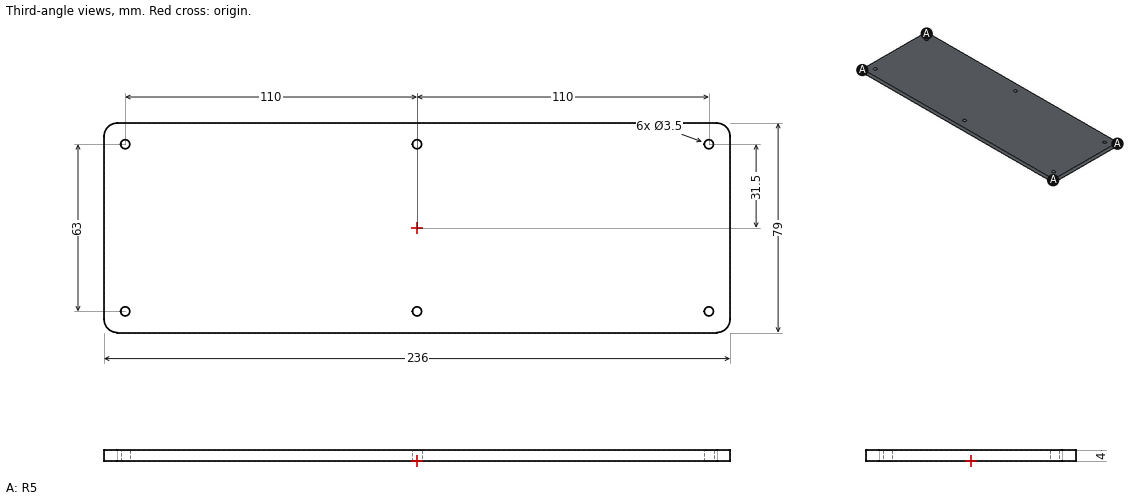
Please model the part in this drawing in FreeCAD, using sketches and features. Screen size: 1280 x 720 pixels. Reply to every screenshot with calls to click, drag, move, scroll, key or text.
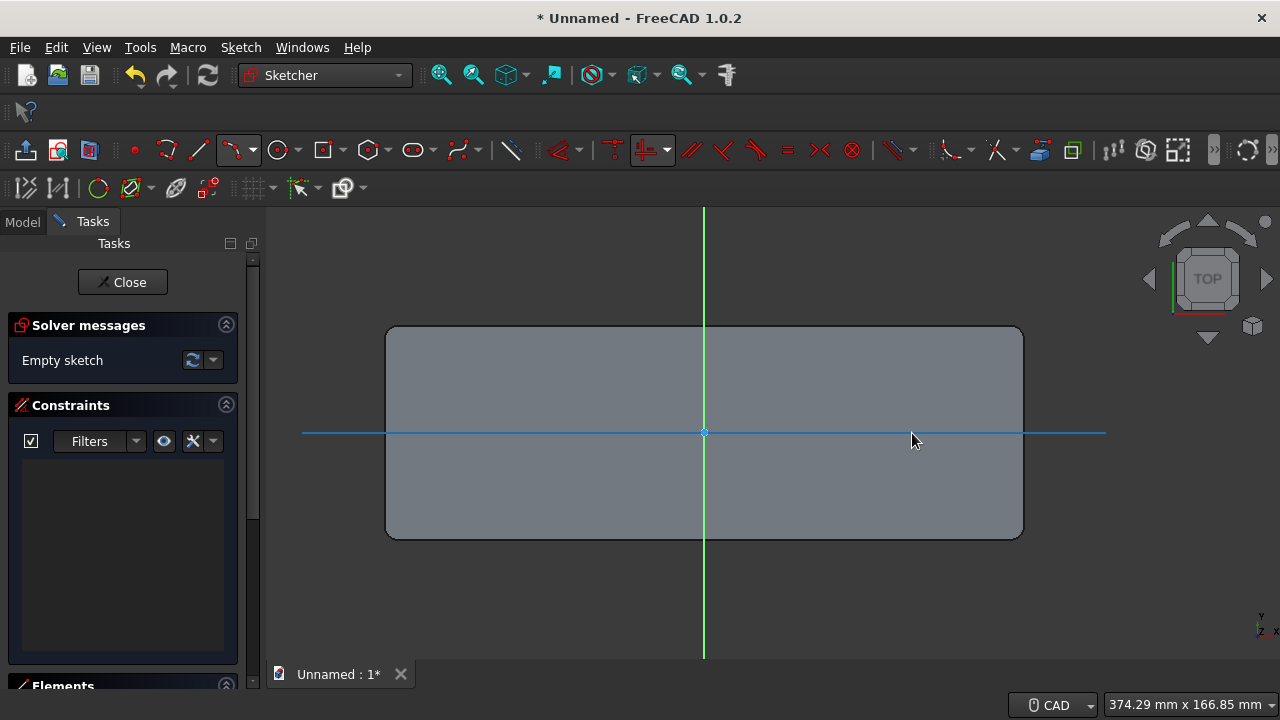
click(278, 150)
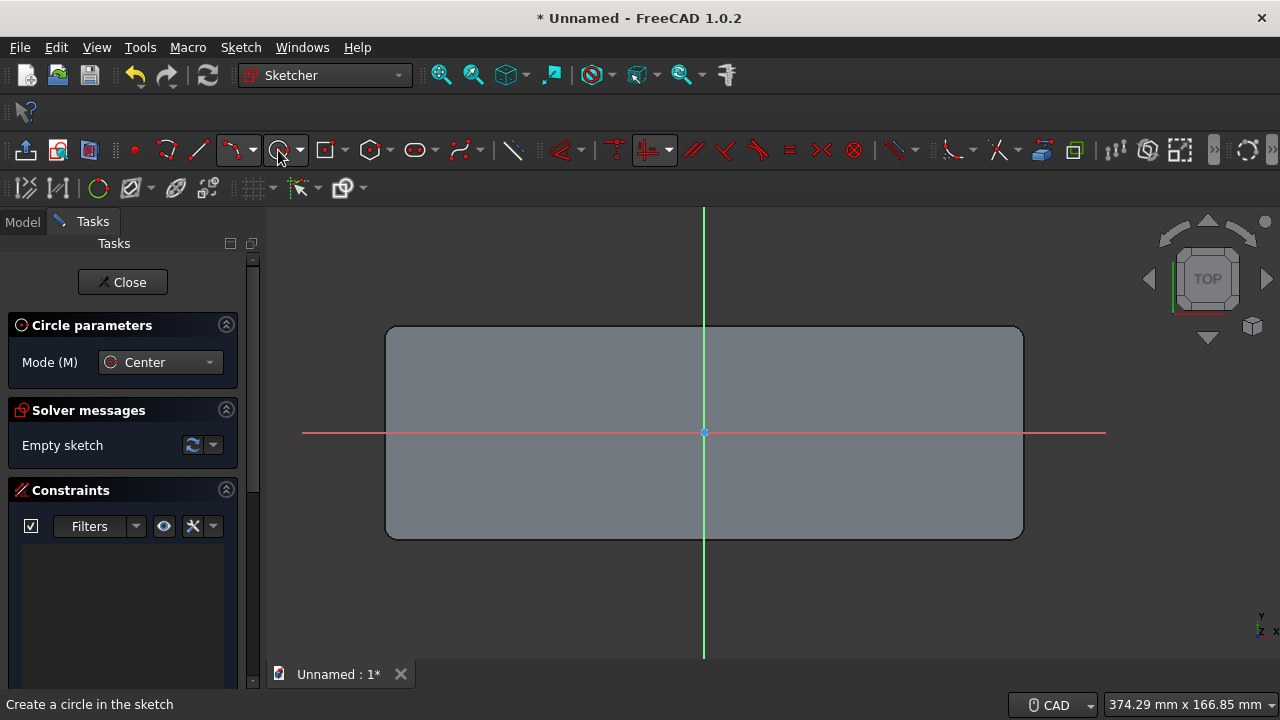
scroll(1002, 347, up, 8)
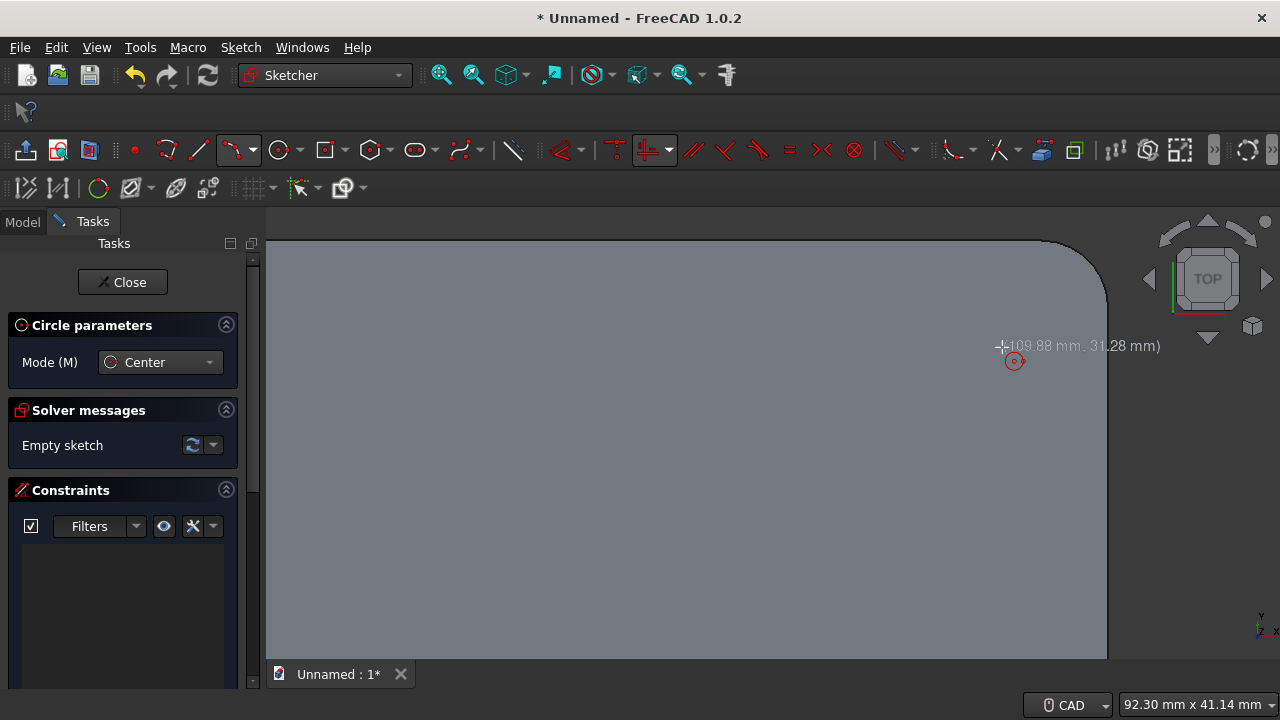
scroll(1003, 348, down, 8)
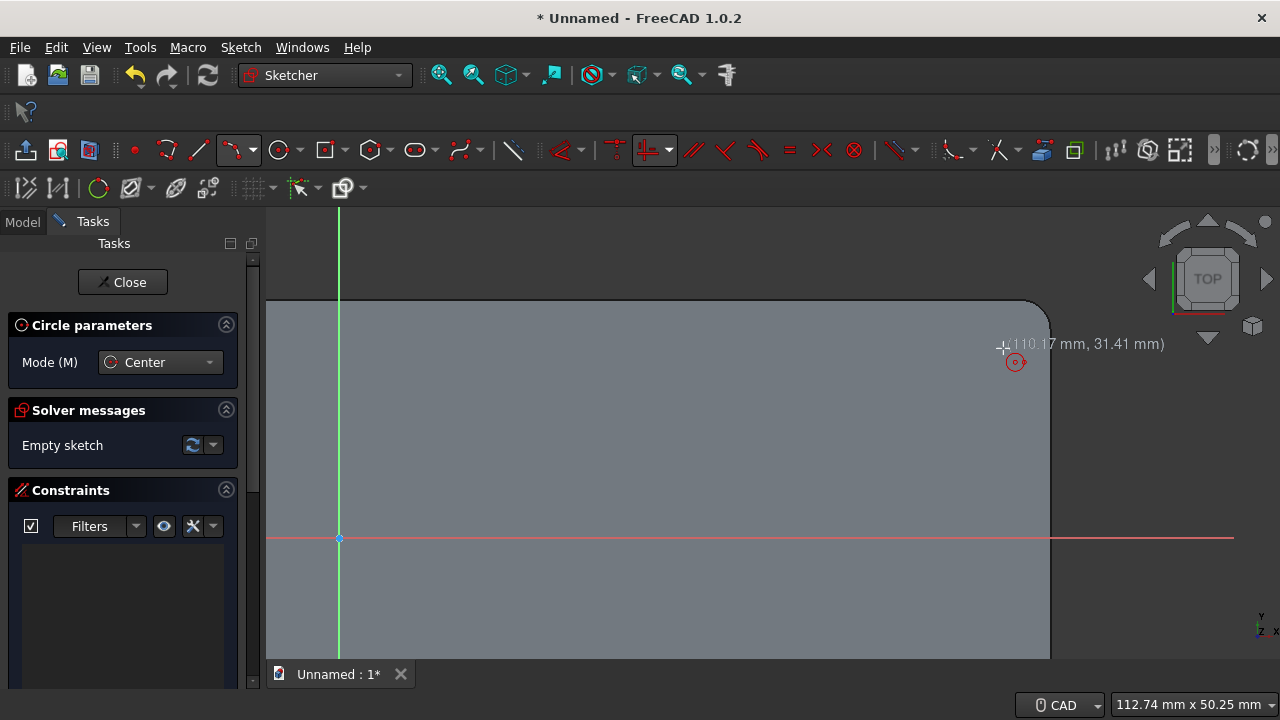
click(1003, 348)
move(1006, 345)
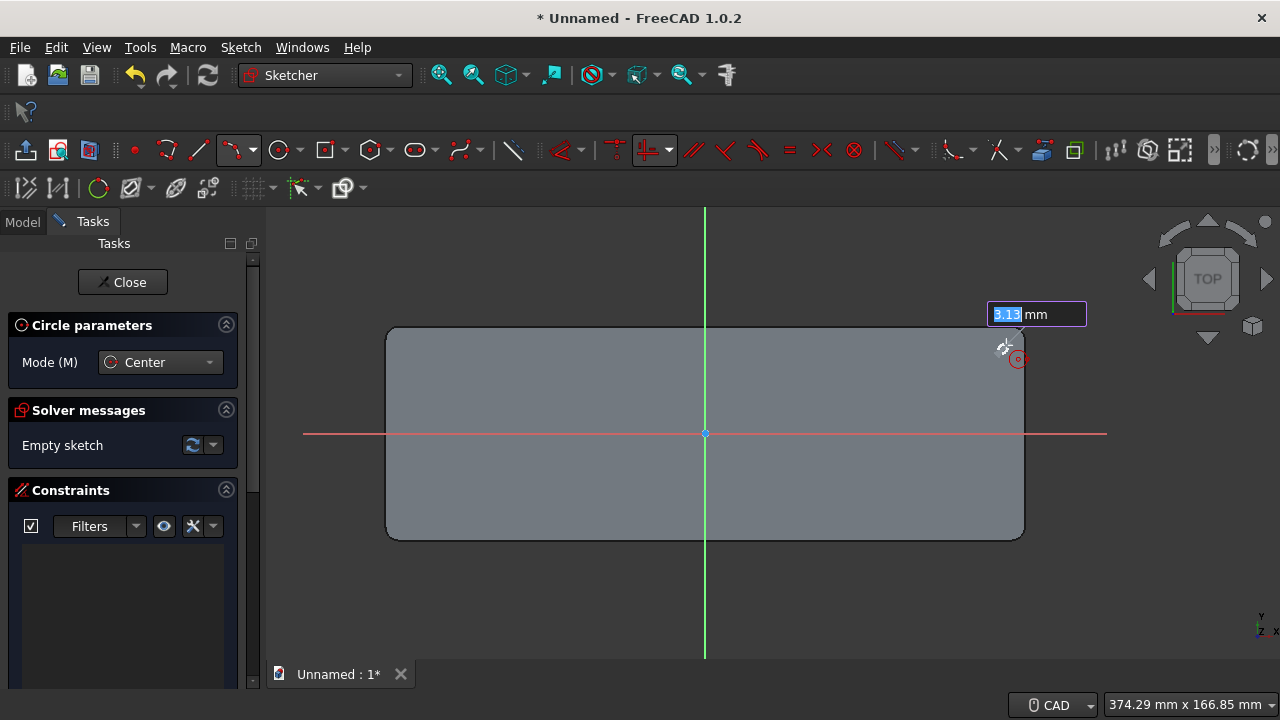
text(3.5)
key(Return)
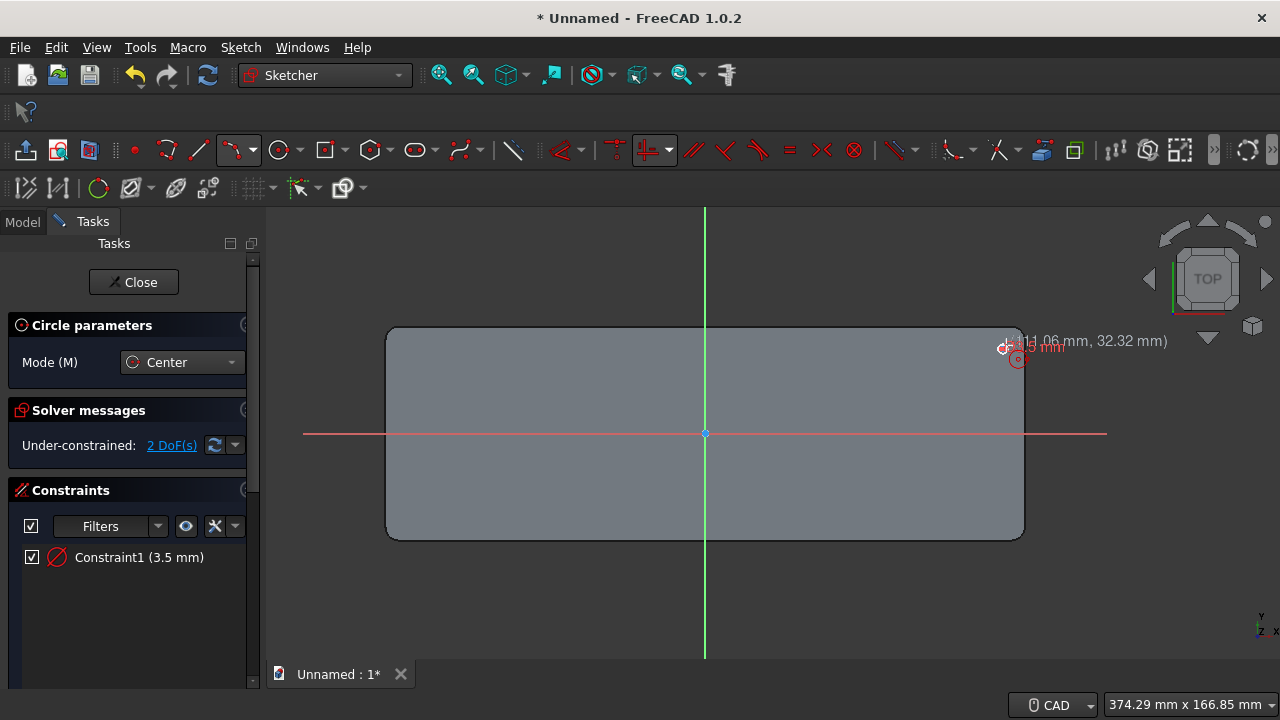
scroll(407, 348, up, 8)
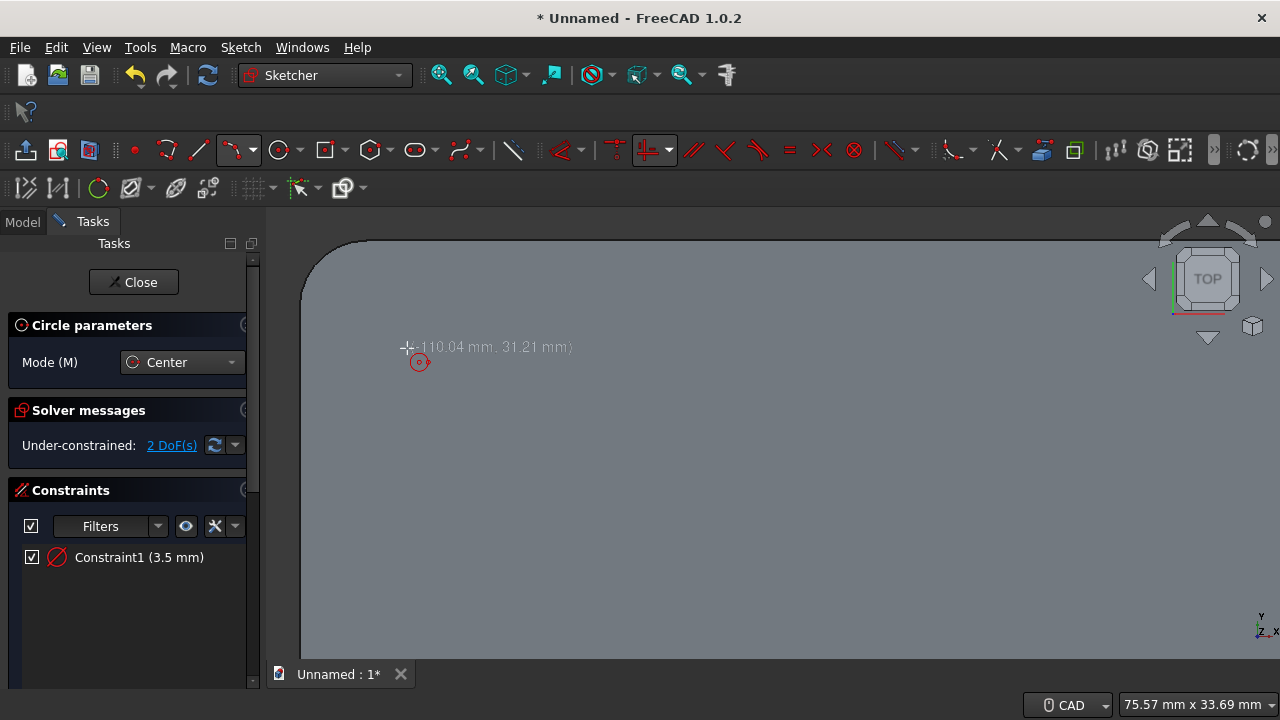
scroll(406, 348, down, 8)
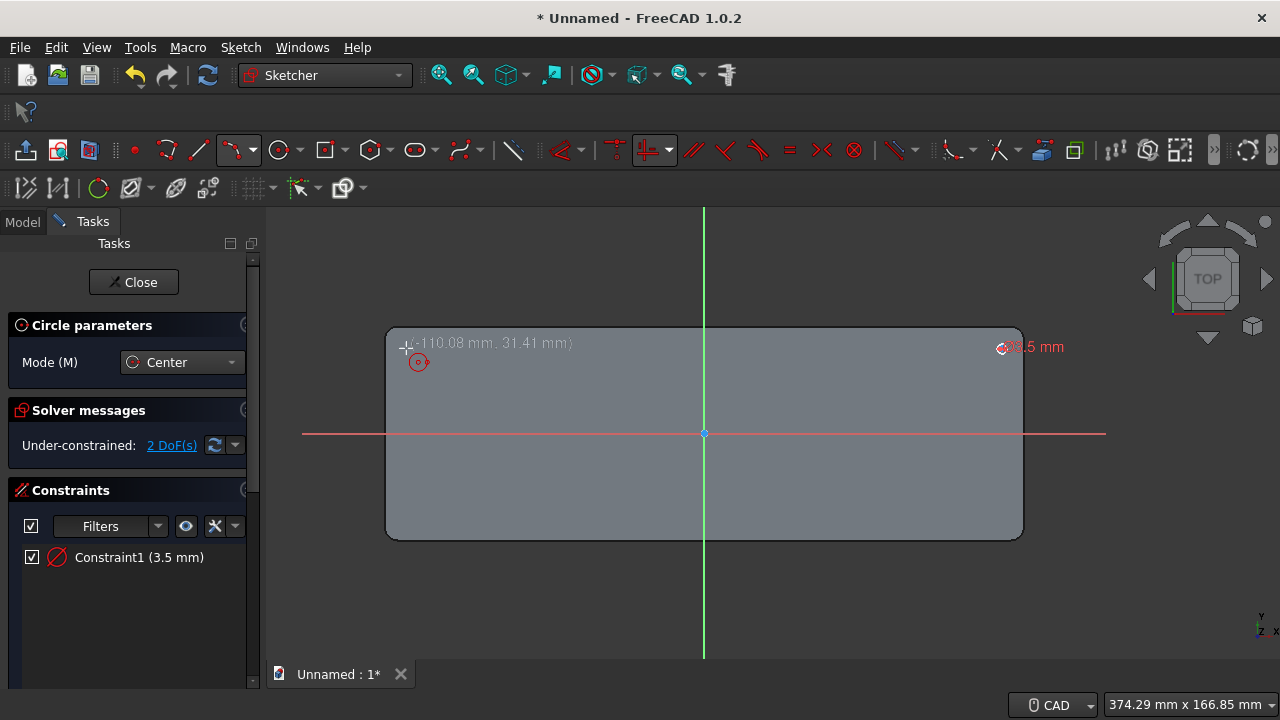
click(406, 348)
move(410, 345)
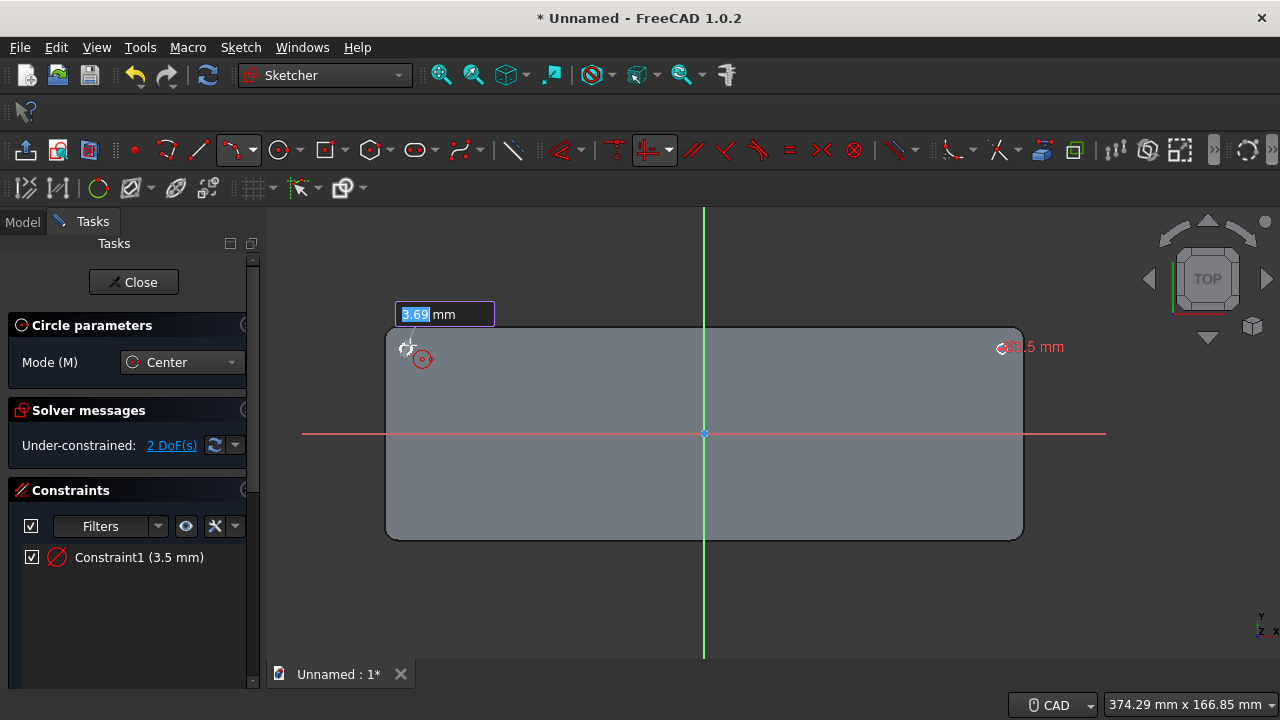
text(3.5)
key(Return)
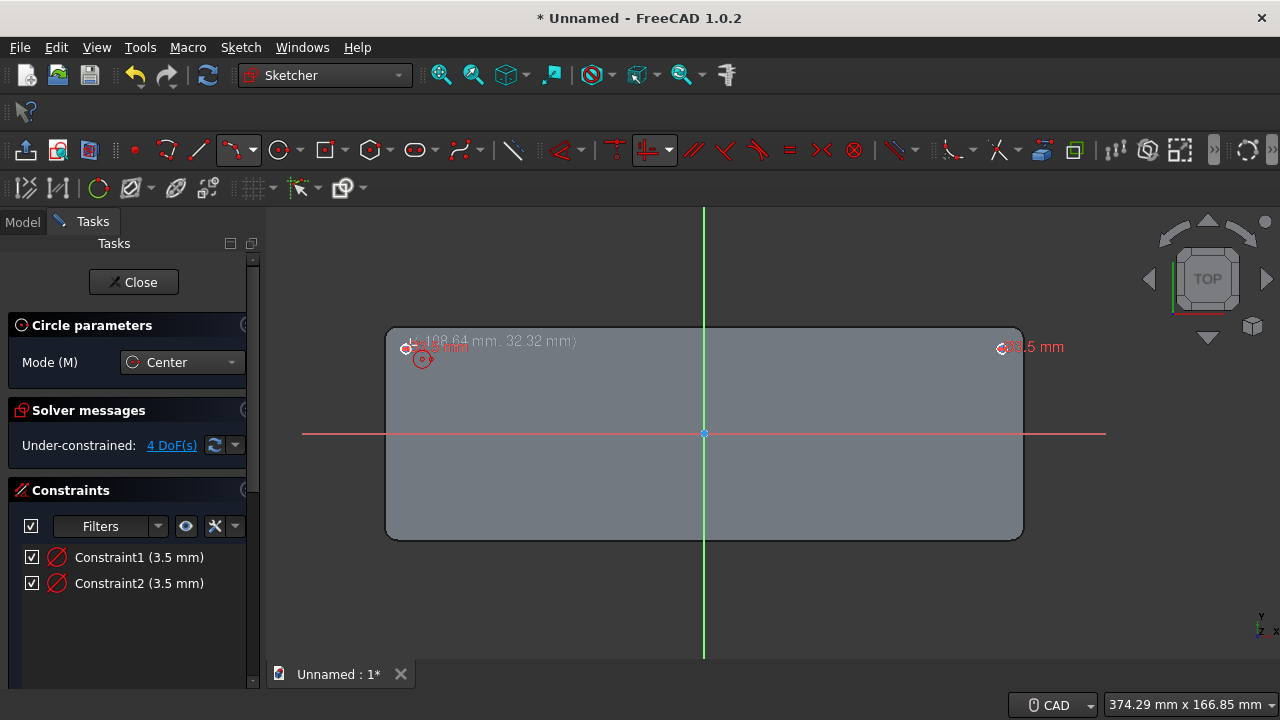
scroll(406, 519, up, 8)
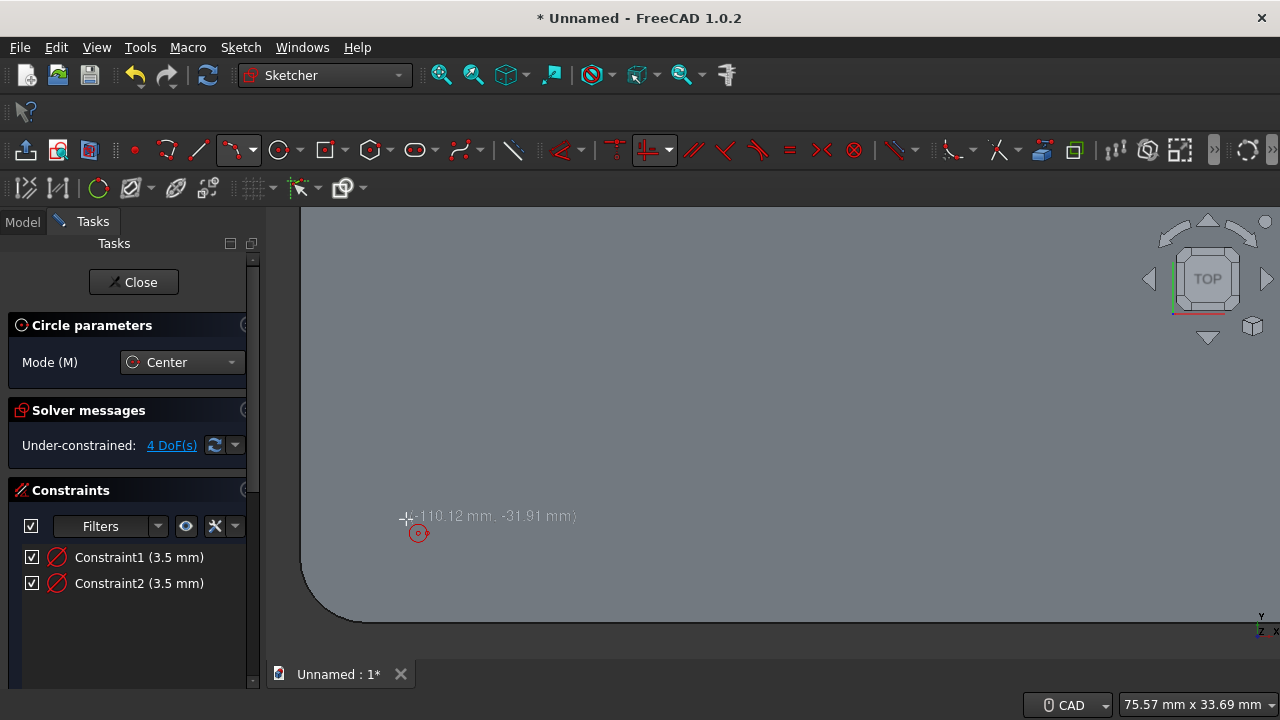
scroll(406, 519, down, 8)